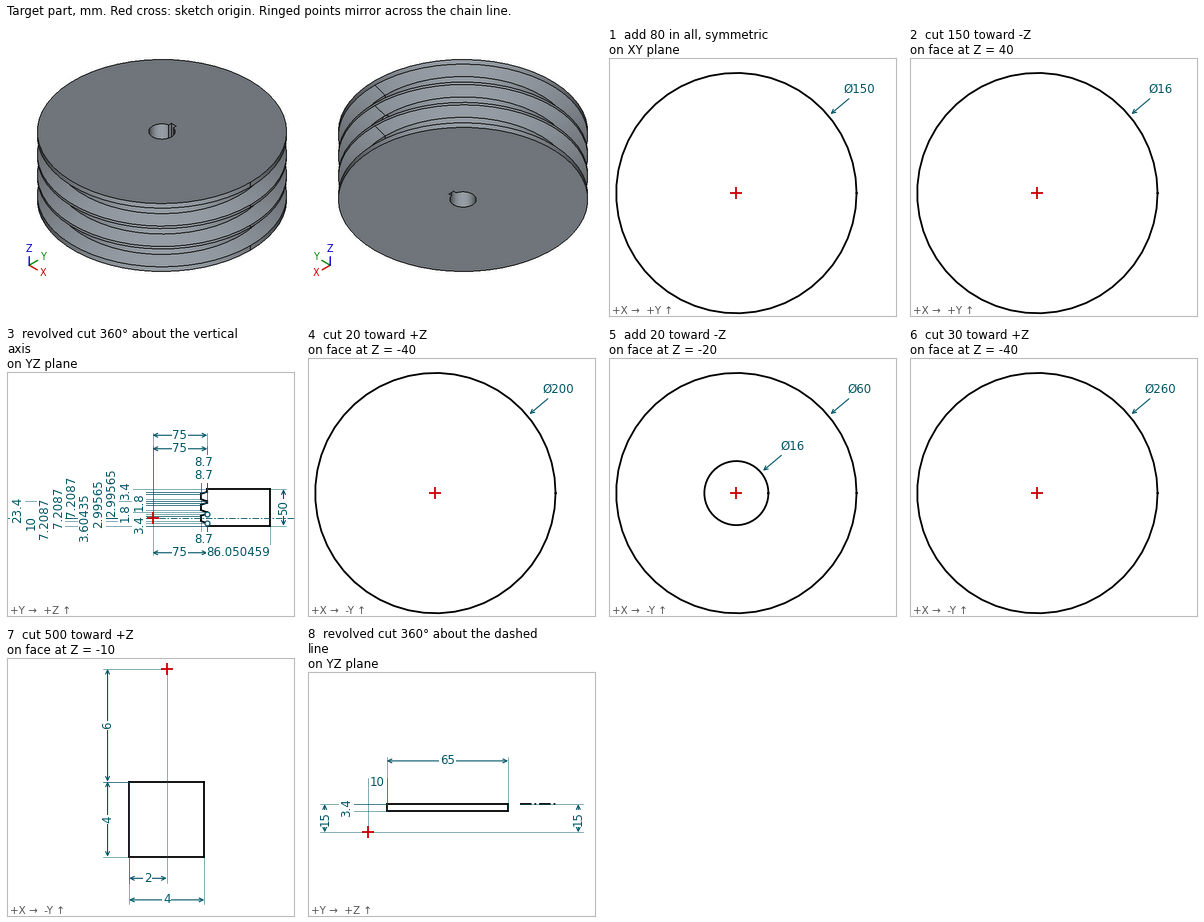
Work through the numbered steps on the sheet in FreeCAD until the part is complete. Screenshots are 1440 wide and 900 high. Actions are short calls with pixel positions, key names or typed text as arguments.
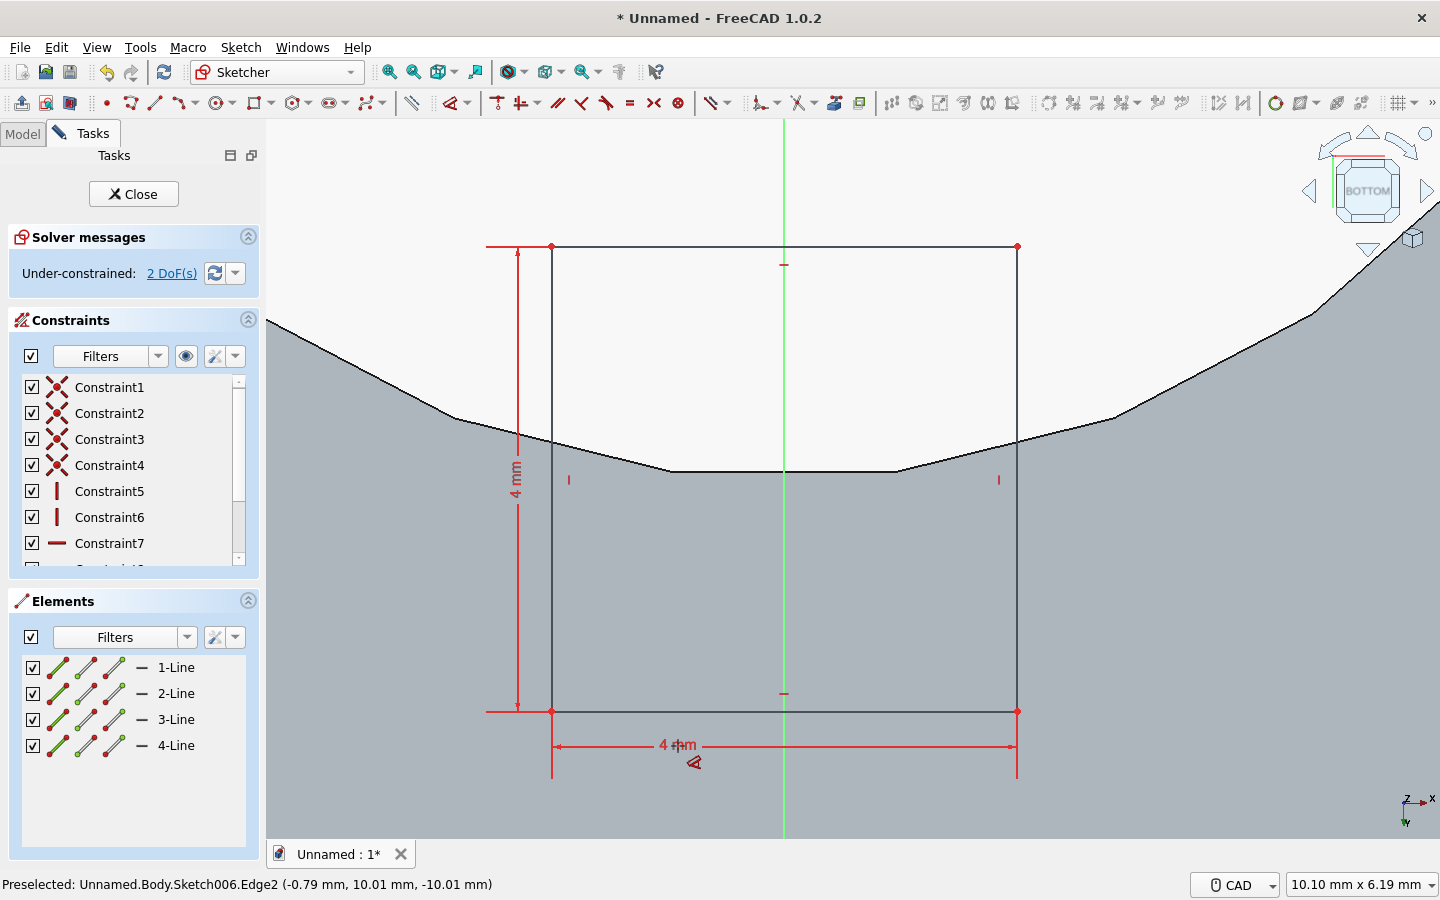
click(552, 247)
click(668, 281)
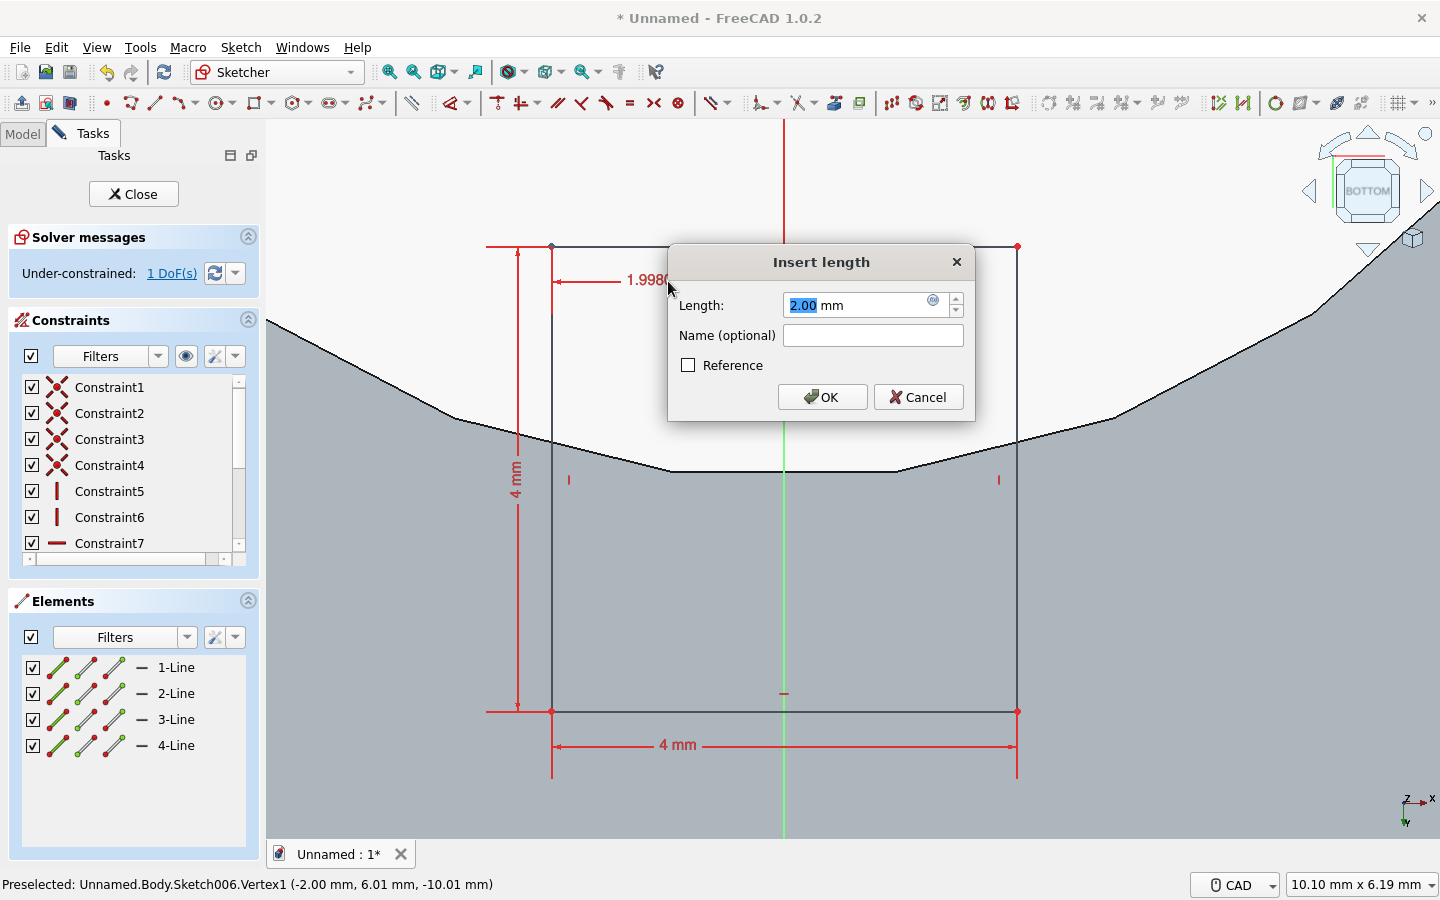
text(2)
key(Return)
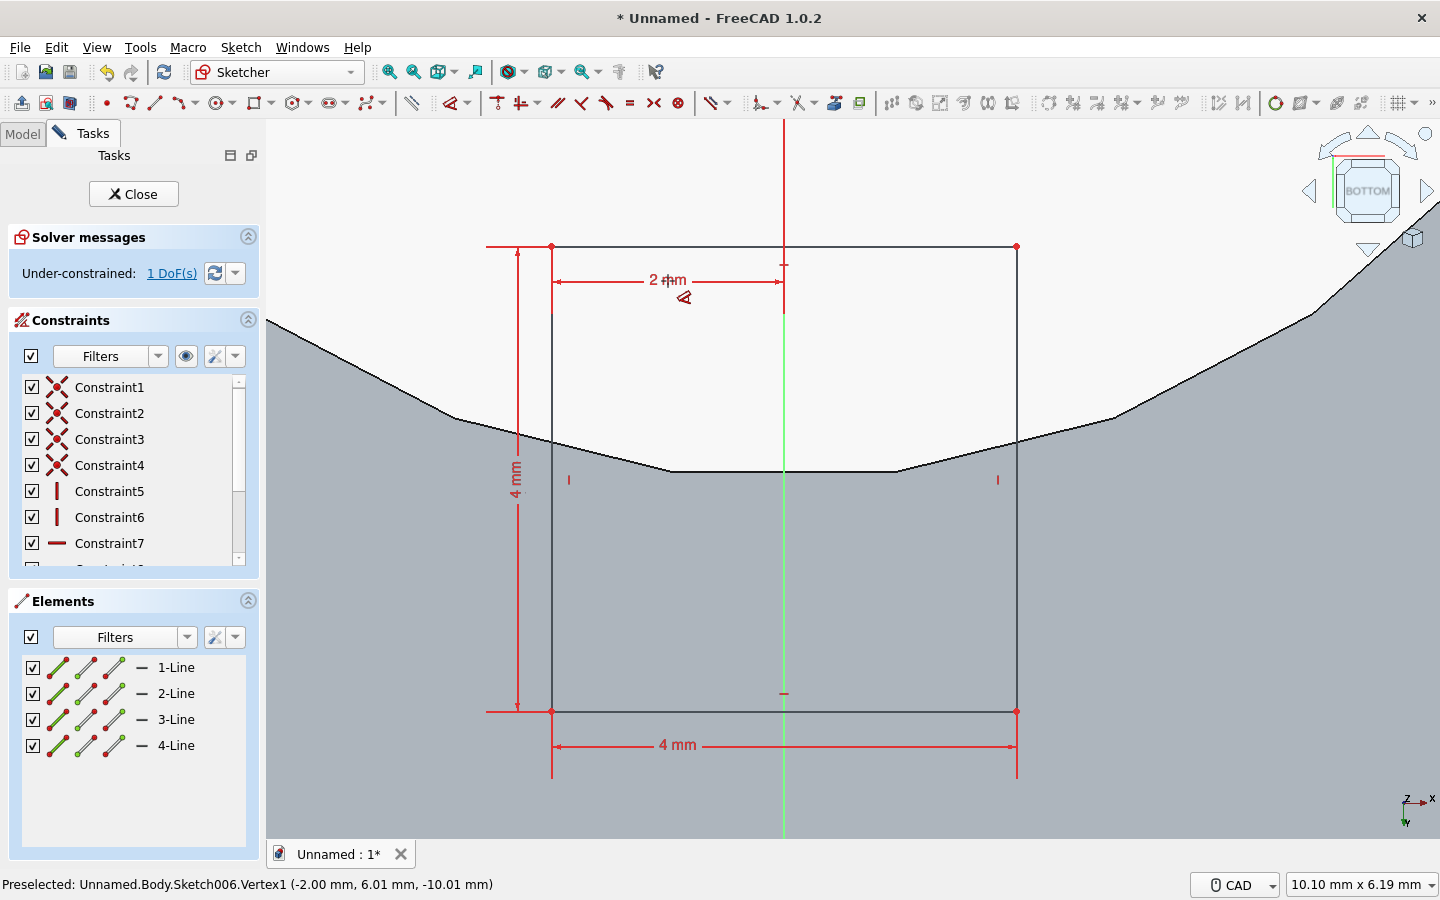
click(552, 247)
click(518, 197)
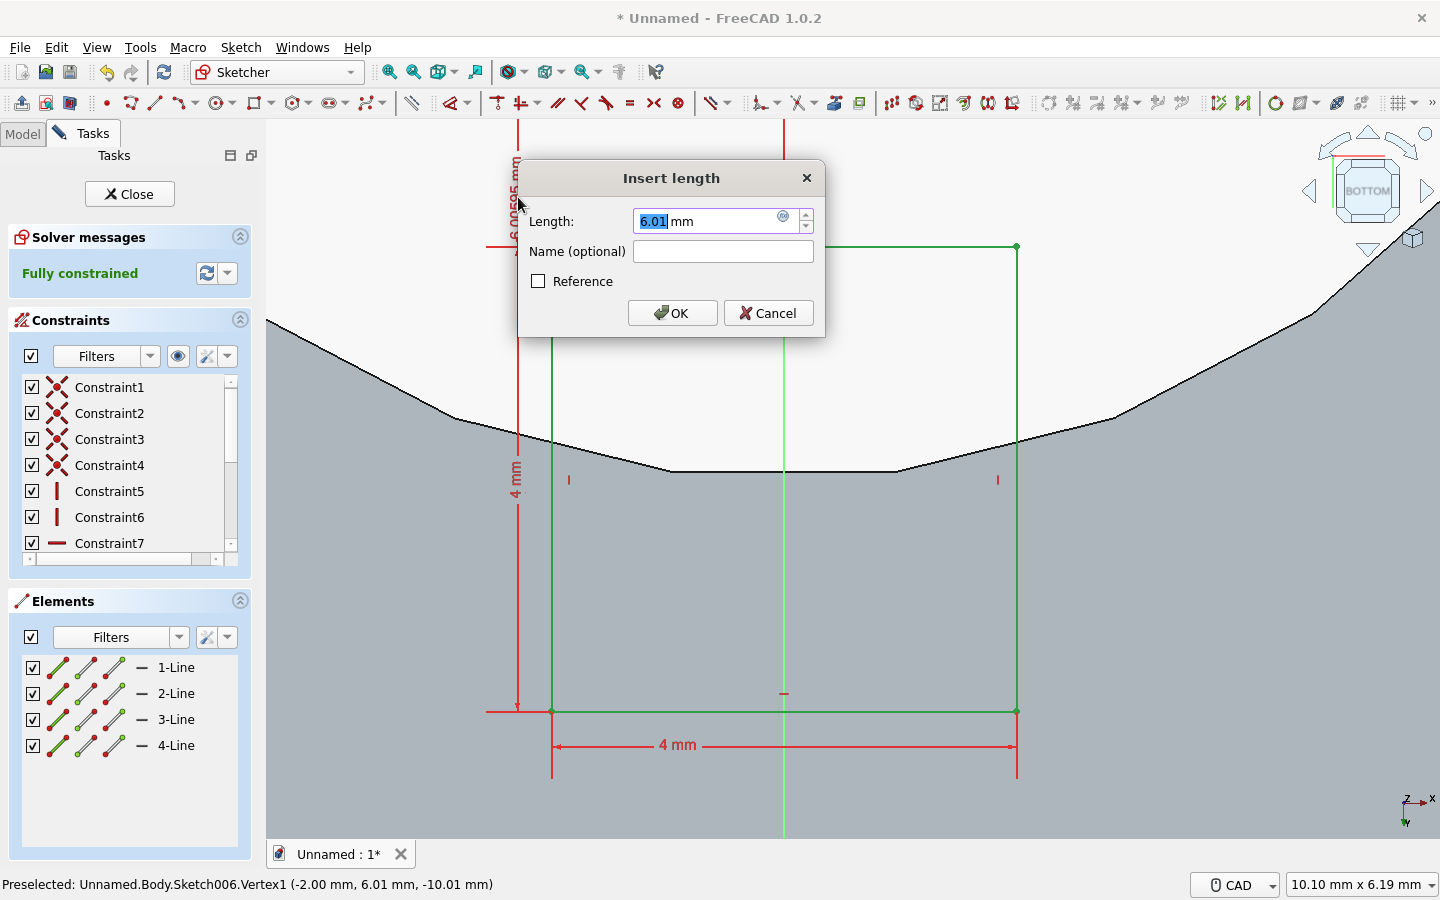
text(6)
key(Return)
key(Escape)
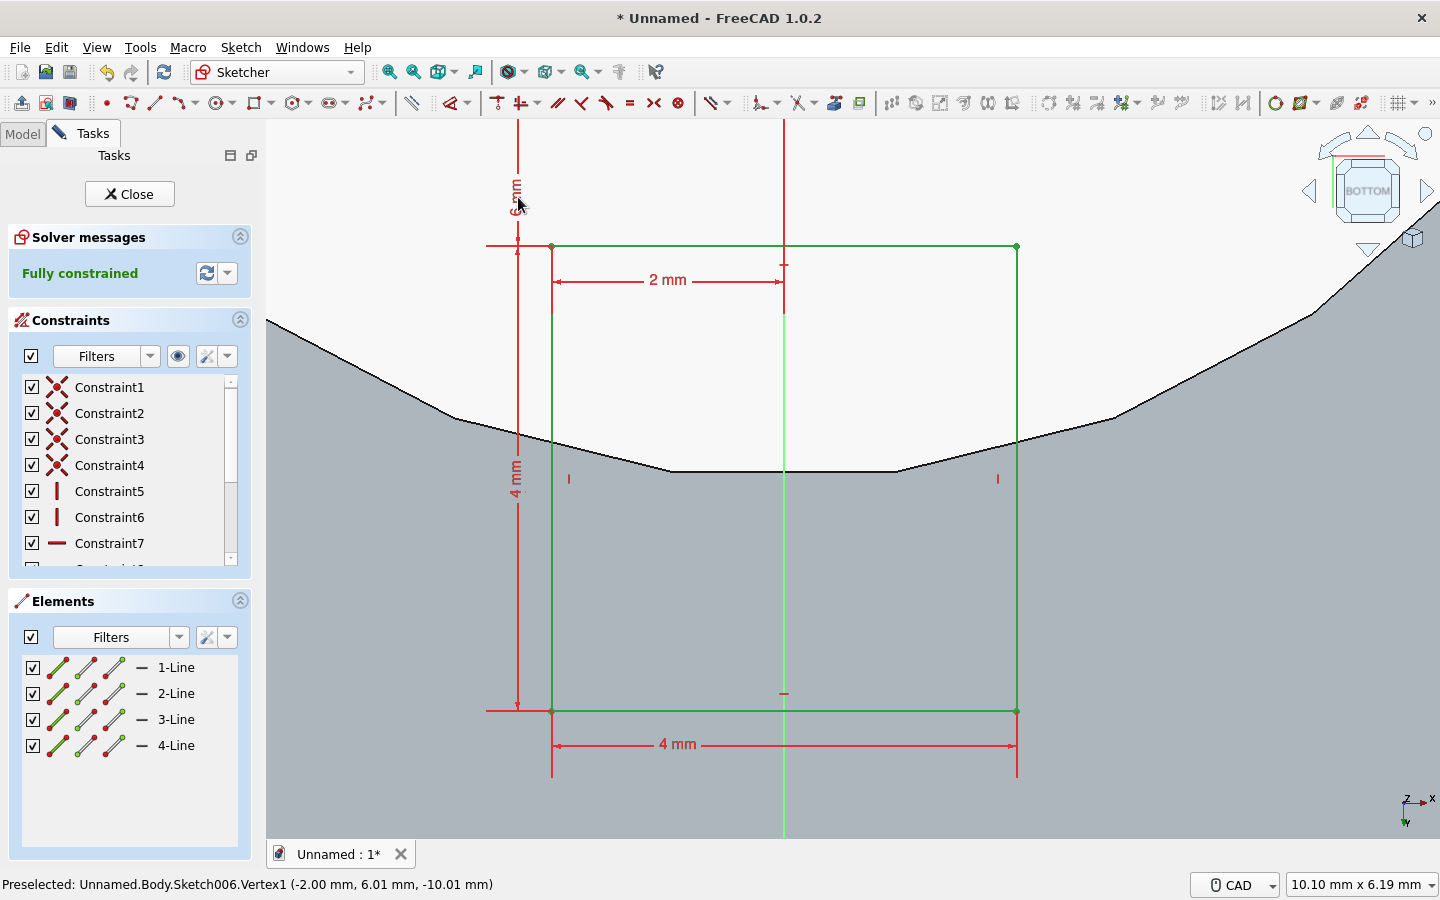
click(130, 194)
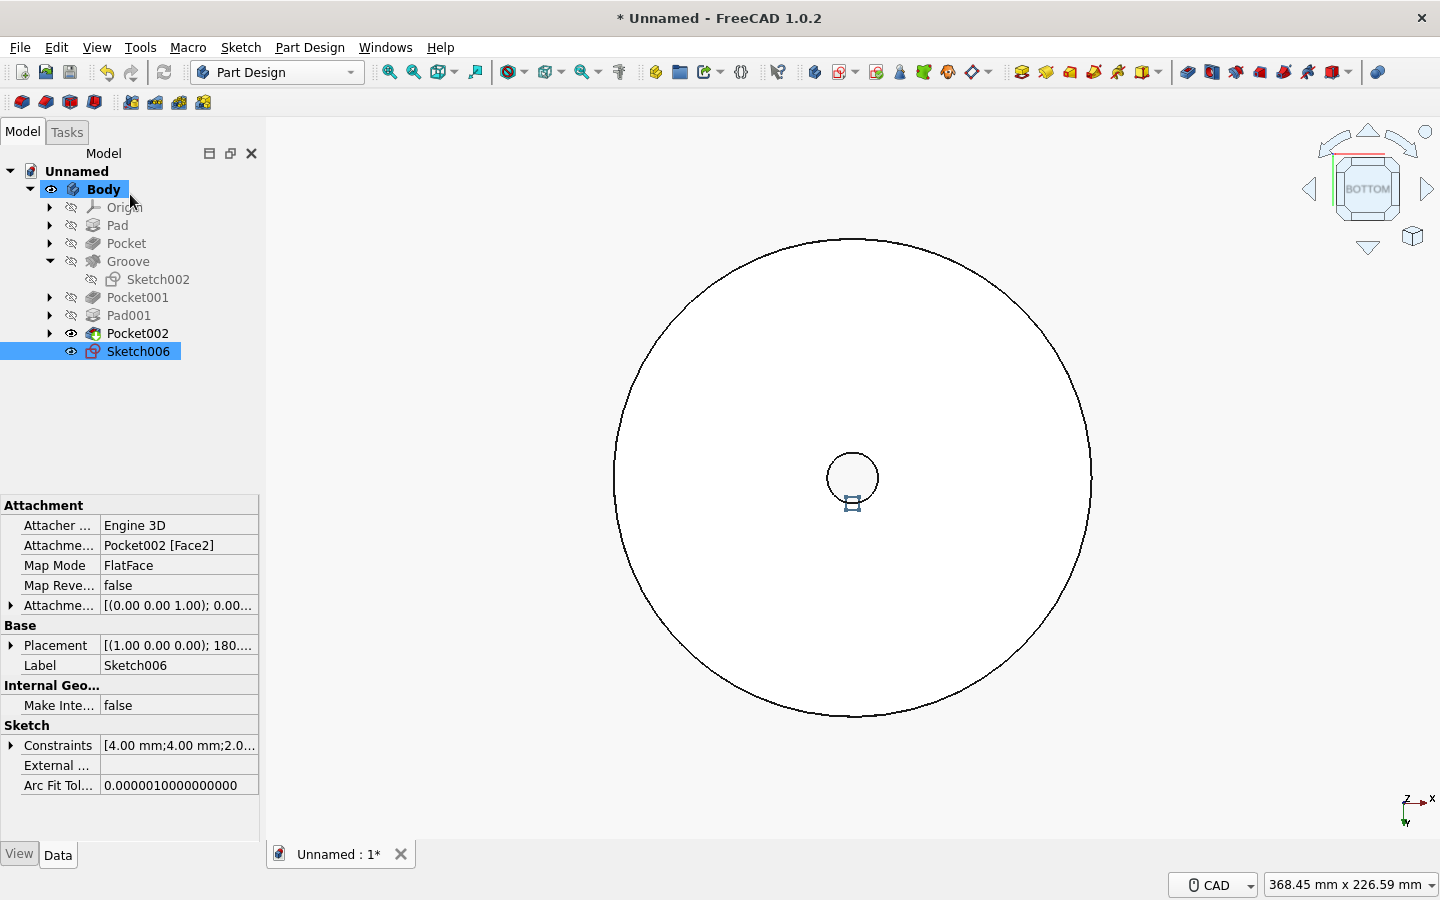
click(1188, 72)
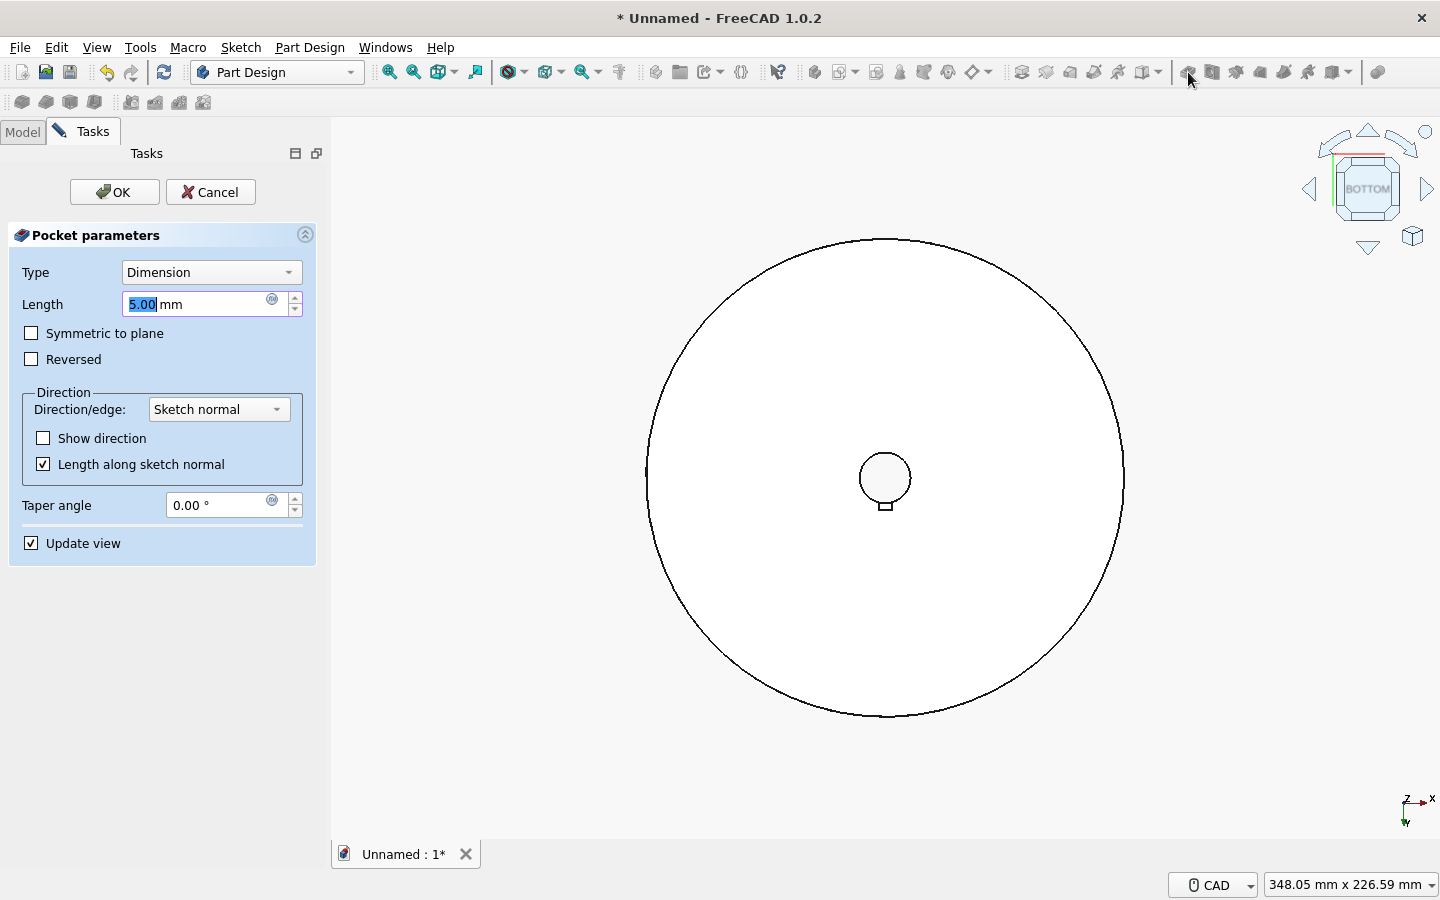
text(500)
key(Tab)